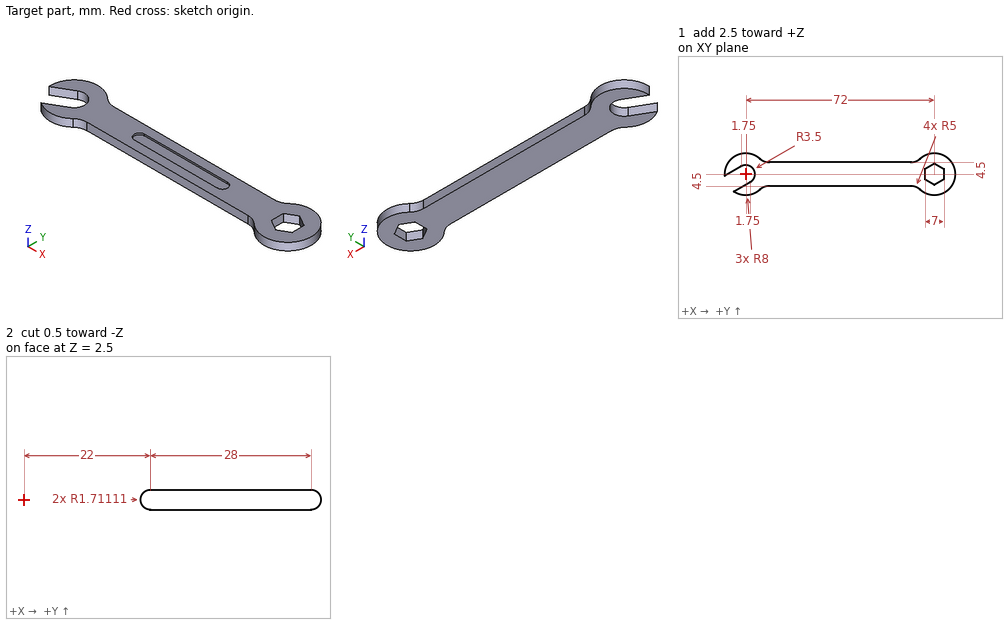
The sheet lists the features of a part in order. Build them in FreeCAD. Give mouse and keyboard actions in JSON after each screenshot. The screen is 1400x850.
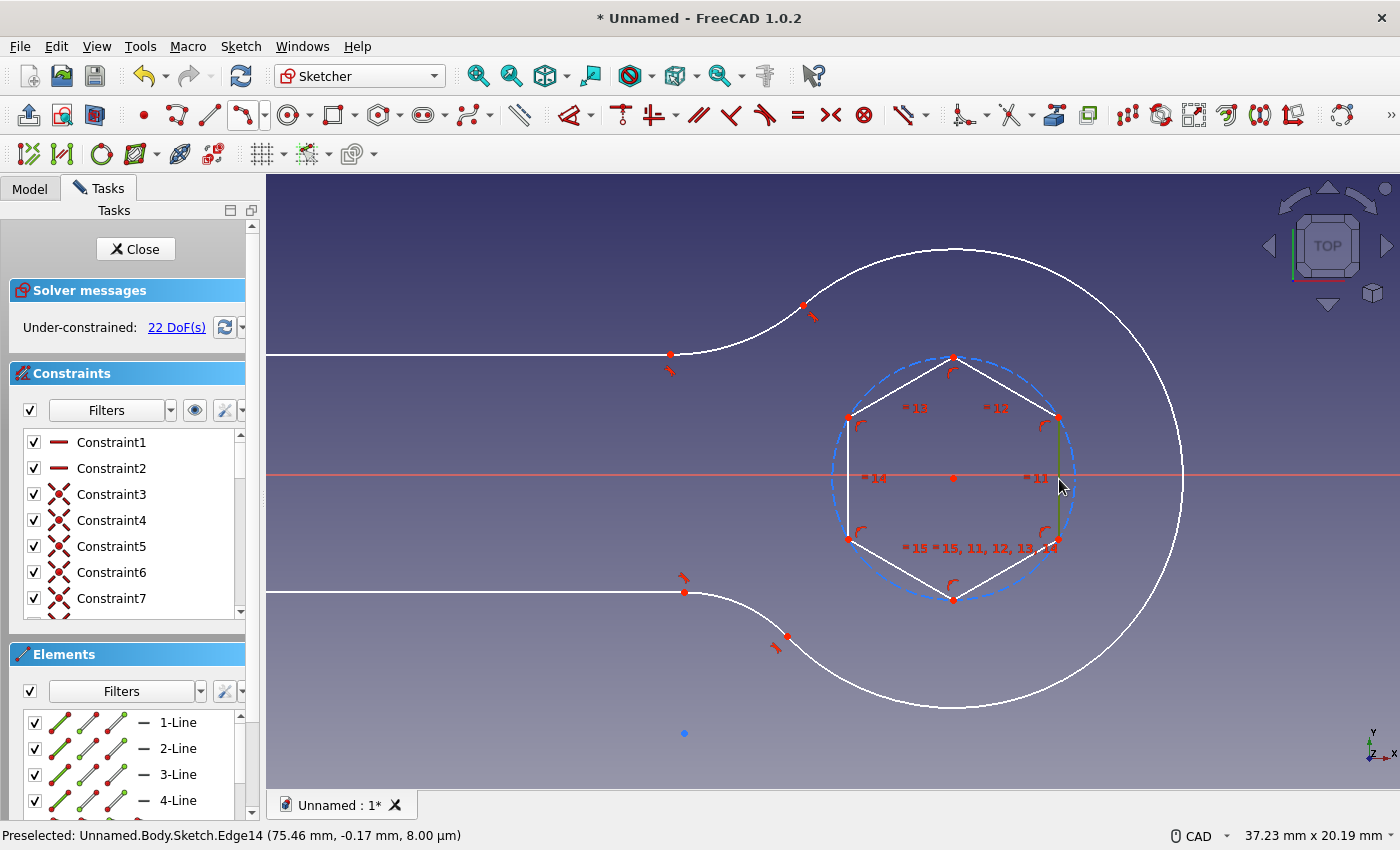
{"action": "left_click", "coordinate": [676, 116]}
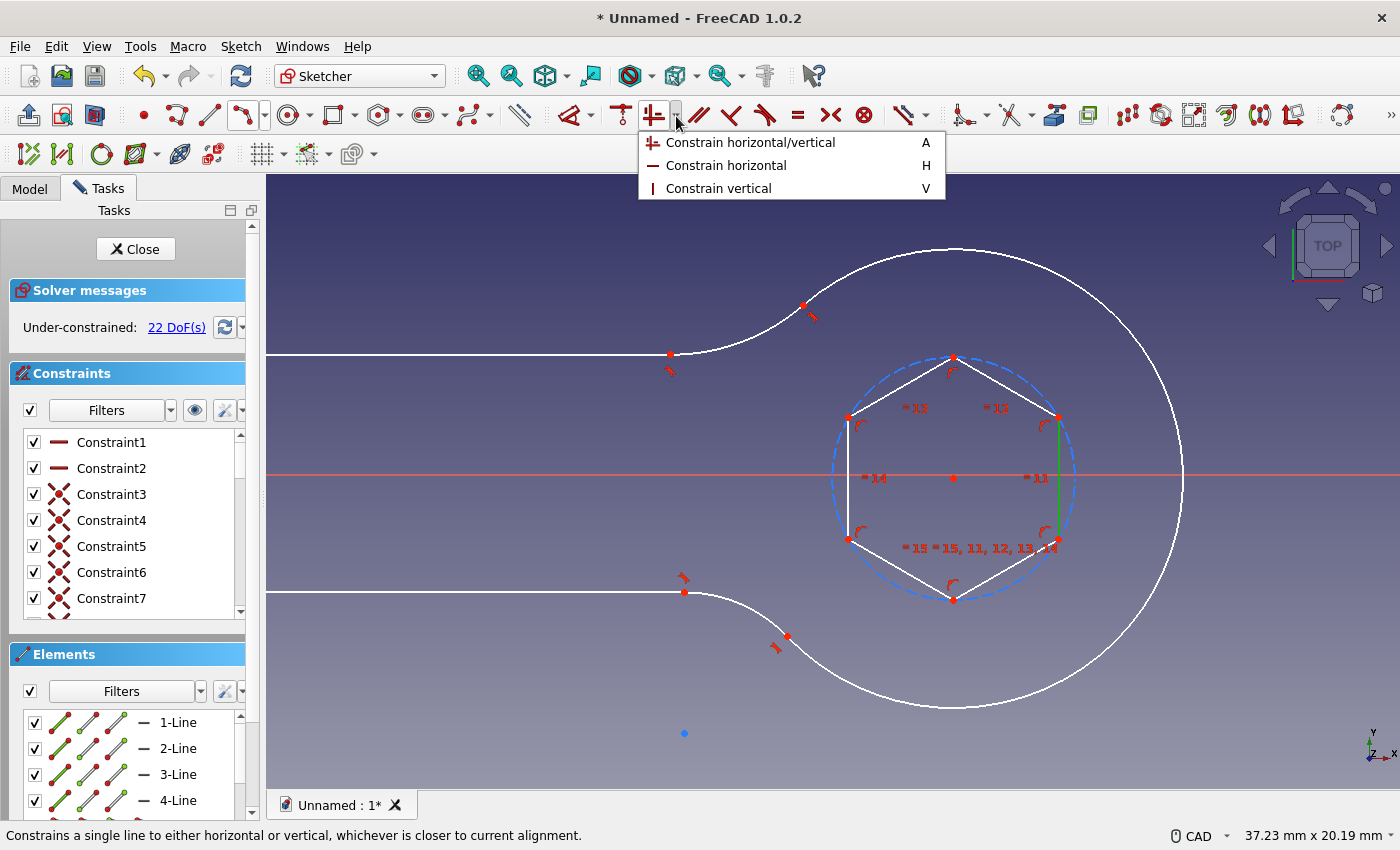
{"action": "left_click", "coordinate": [792, 188]}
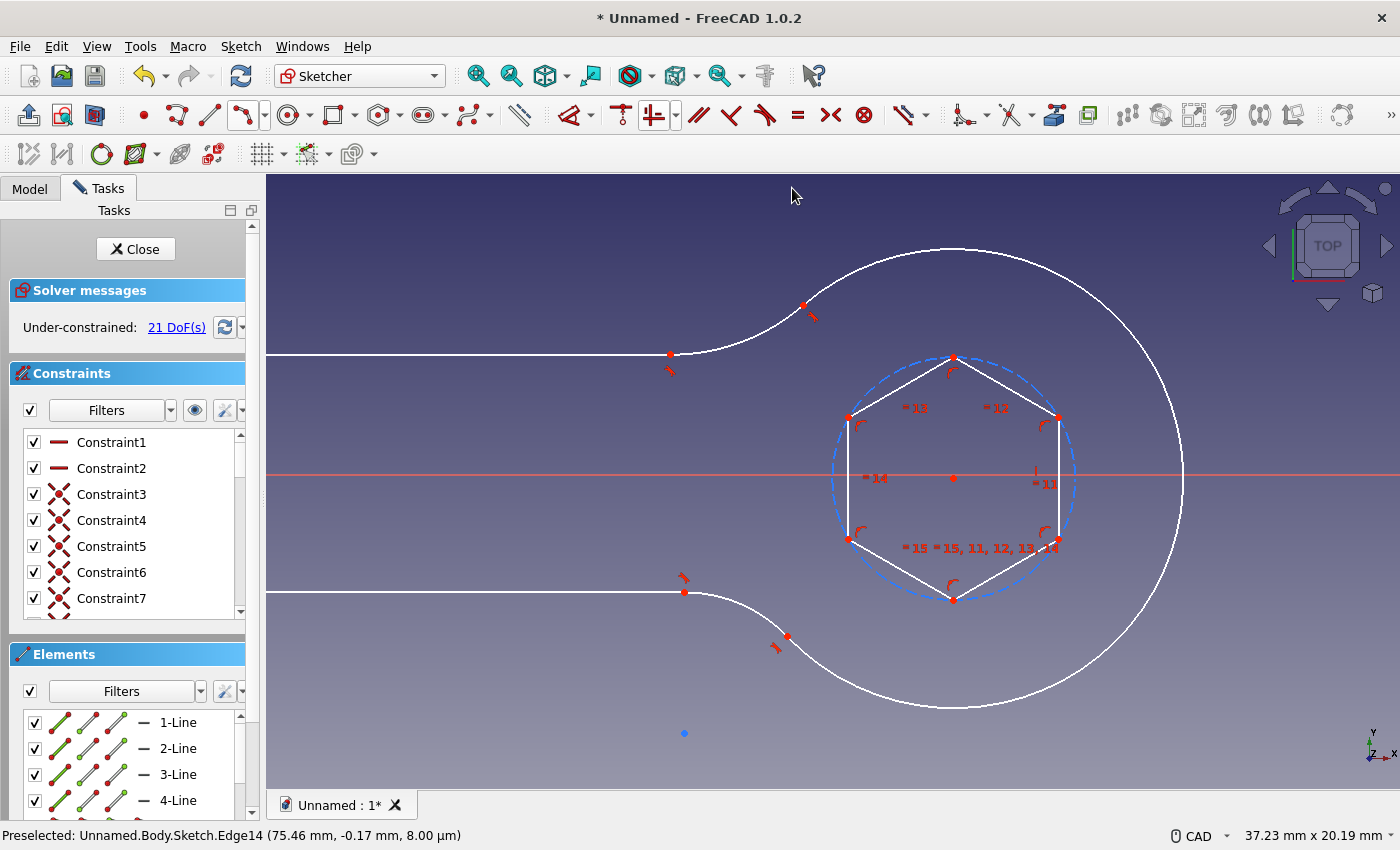
{"action": "scroll", "coordinate": [1061, 480], "scroll_direction": "down", "scroll_amount": 7}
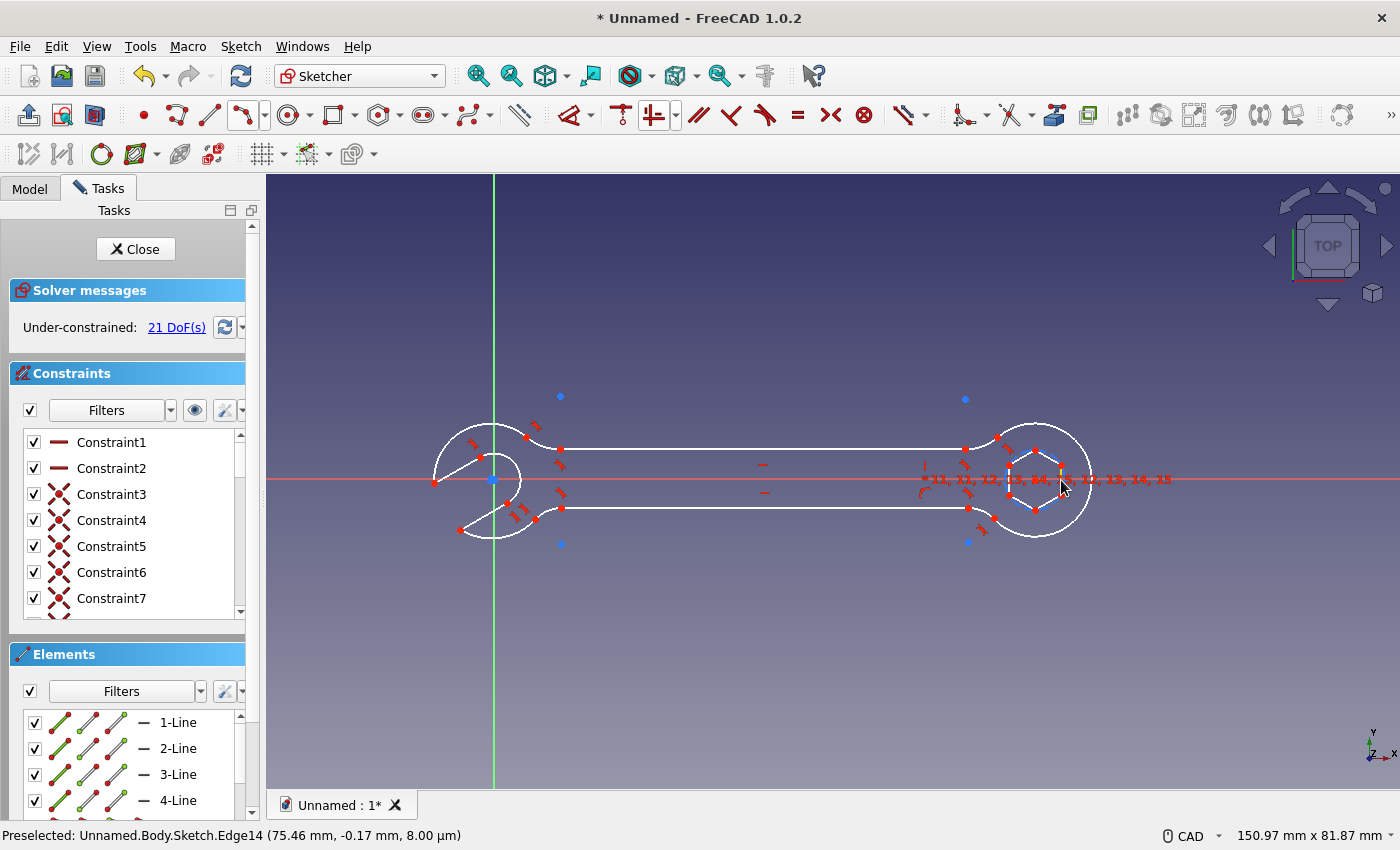
{"action": "scroll", "coordinate": [490, 424], "scroll_direction": "up", "scroll_amount": 7}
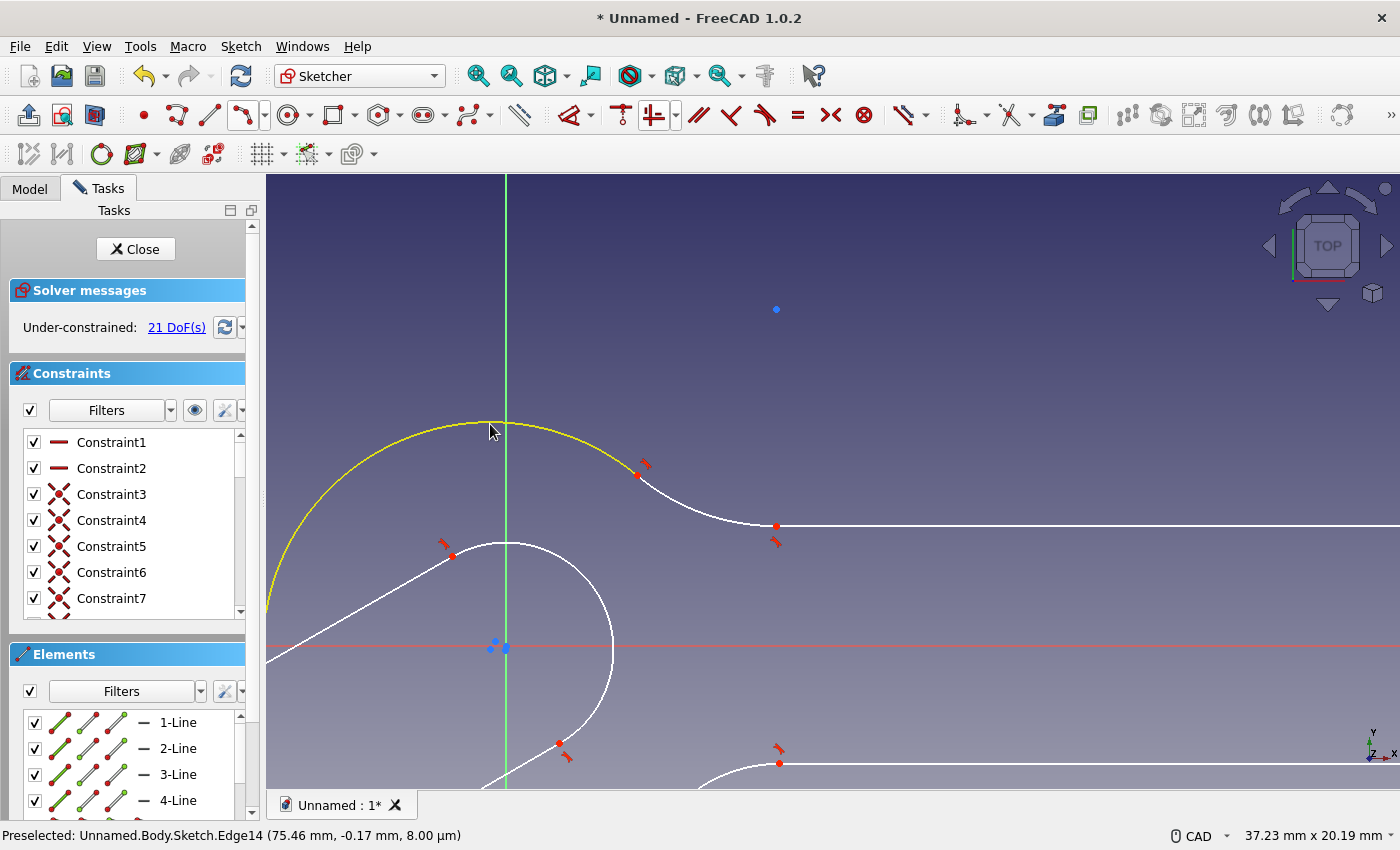
{"action": "left_click", "coordinate": [490, 422]}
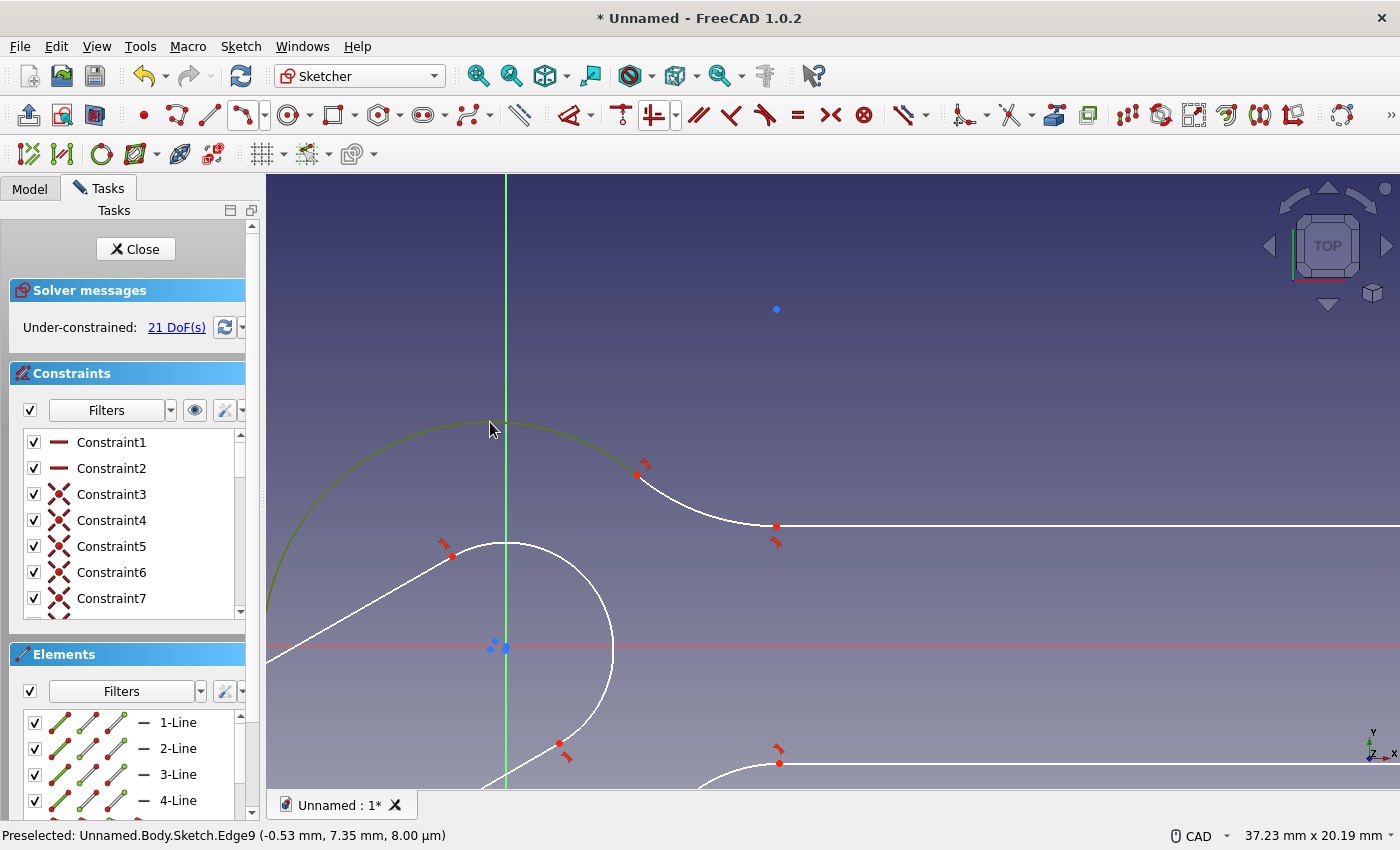
{"action": "left_click", "coordinate": [613, 661]}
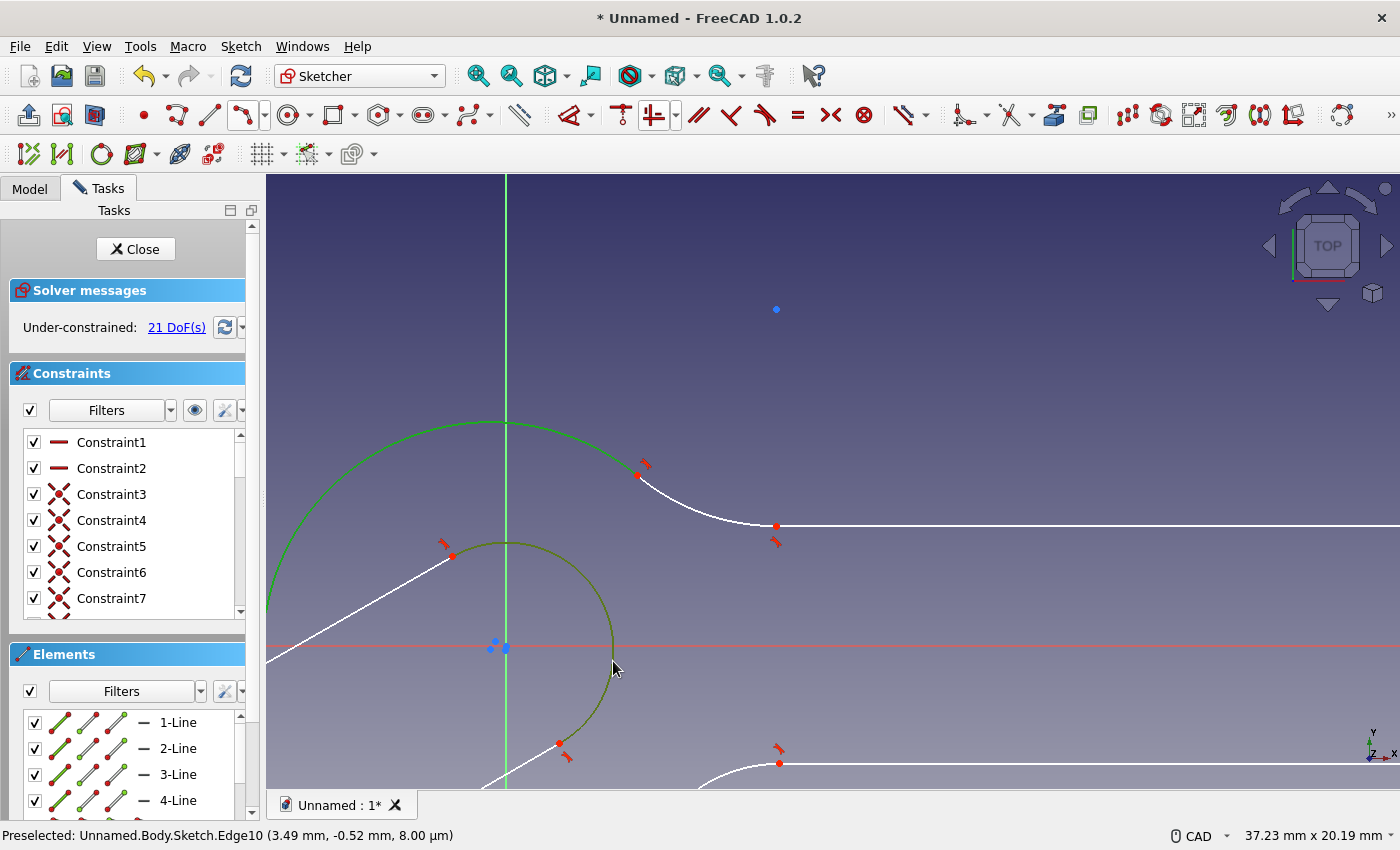
{"action": "left_click", "coordinate": [621, 116]}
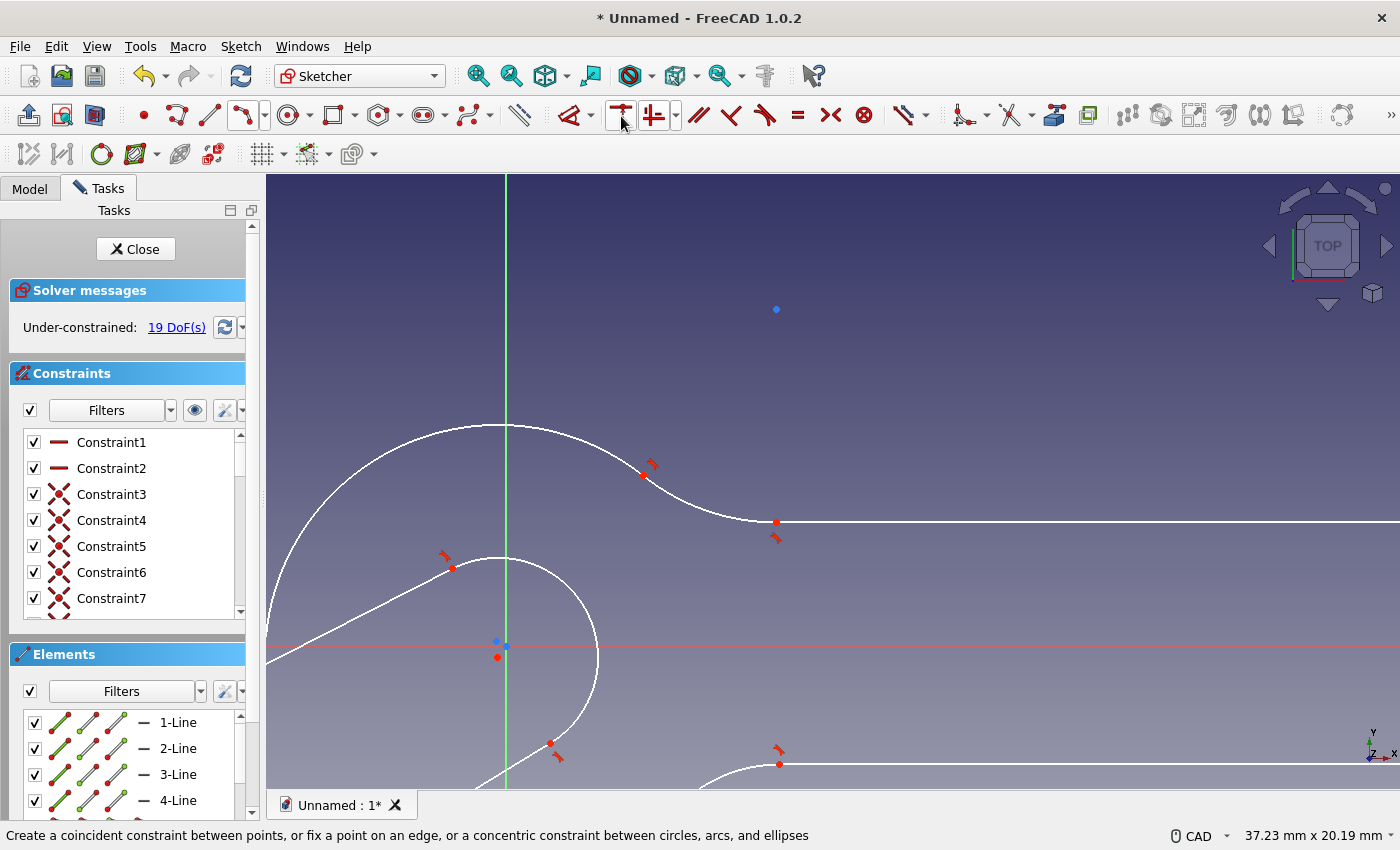
{"action": "scroll", "coordinate": [496, 425], "scroll_direction": "up", "scroll_amount": 2}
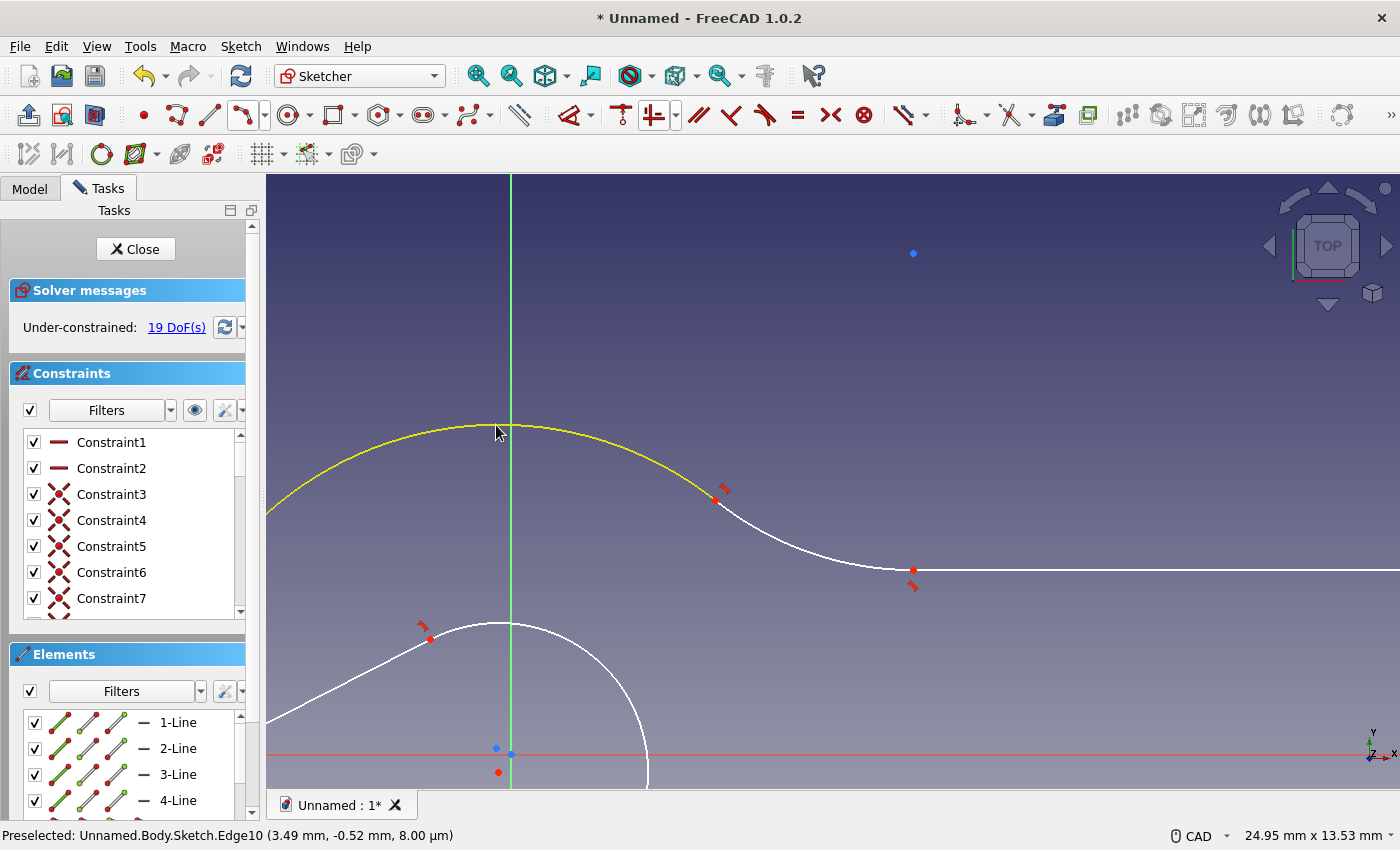
{"action": "left_click", "coordinate": [496, 425]}